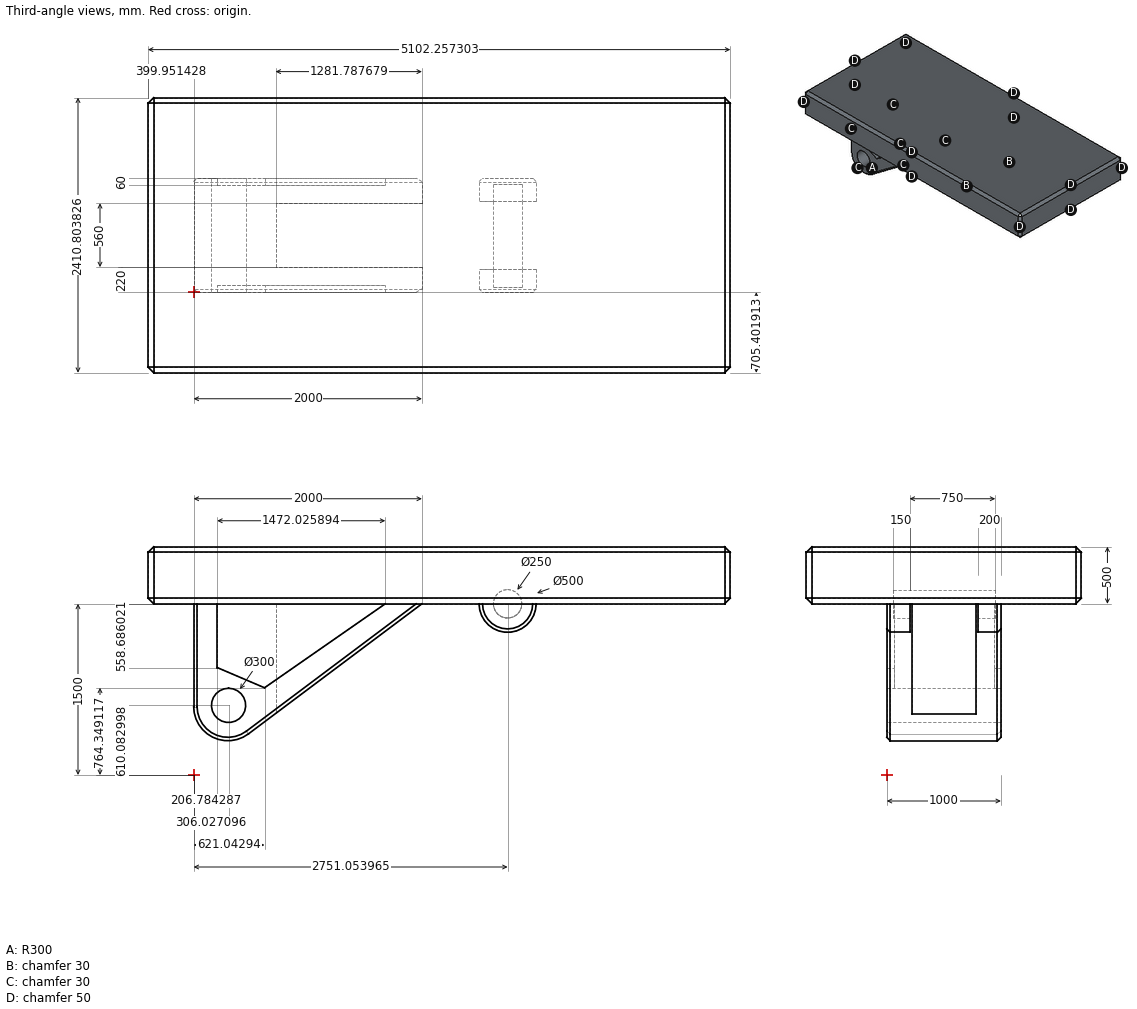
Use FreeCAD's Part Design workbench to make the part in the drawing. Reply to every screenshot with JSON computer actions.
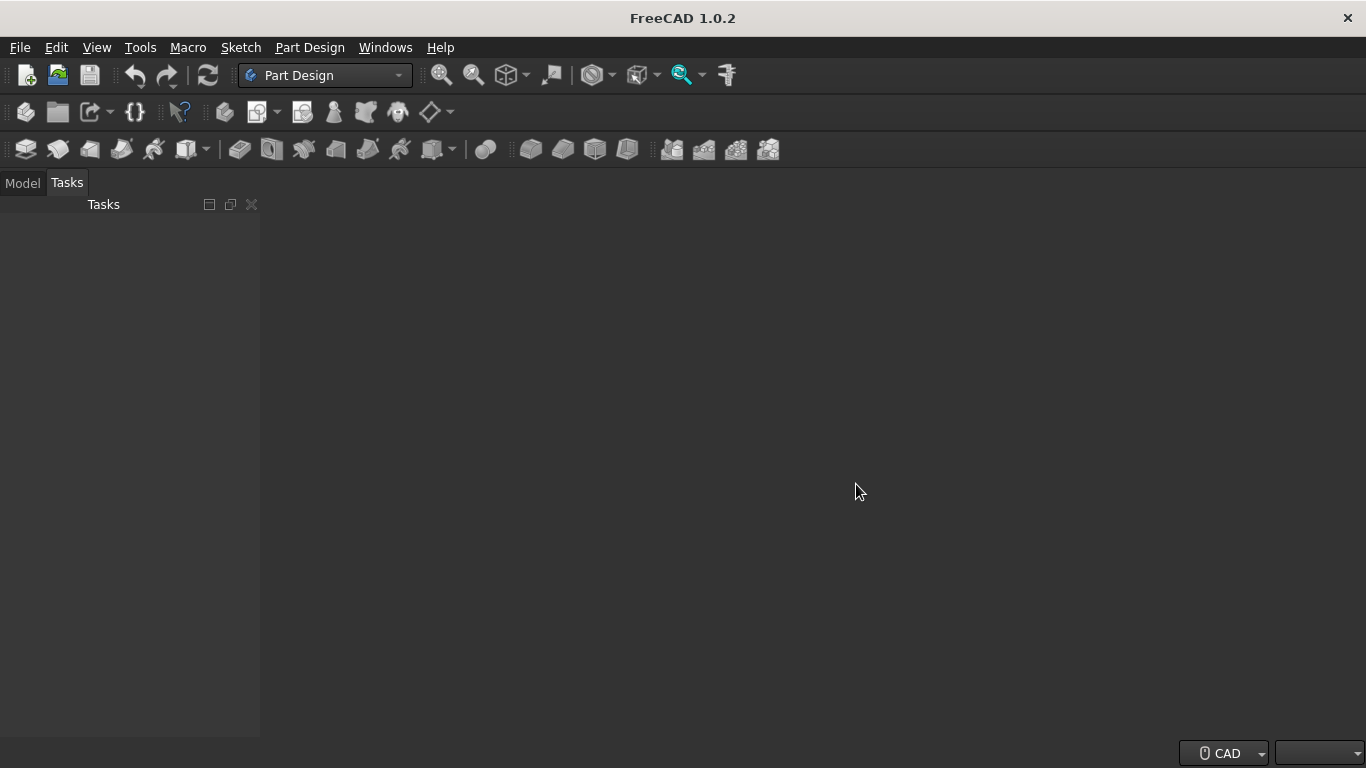
{"action": "left_click", "coordinate": [26, 76]}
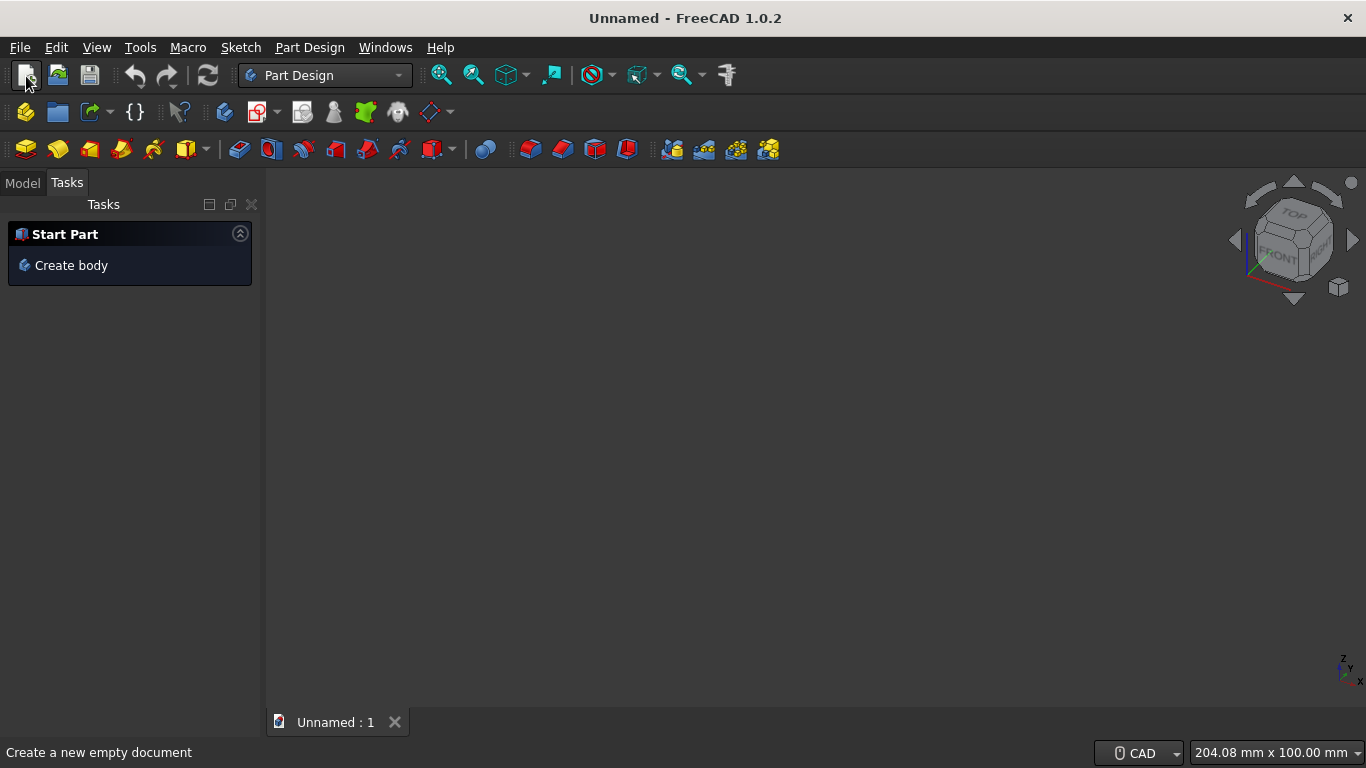
{"action": "left_click", "coordinate": [258, 112]}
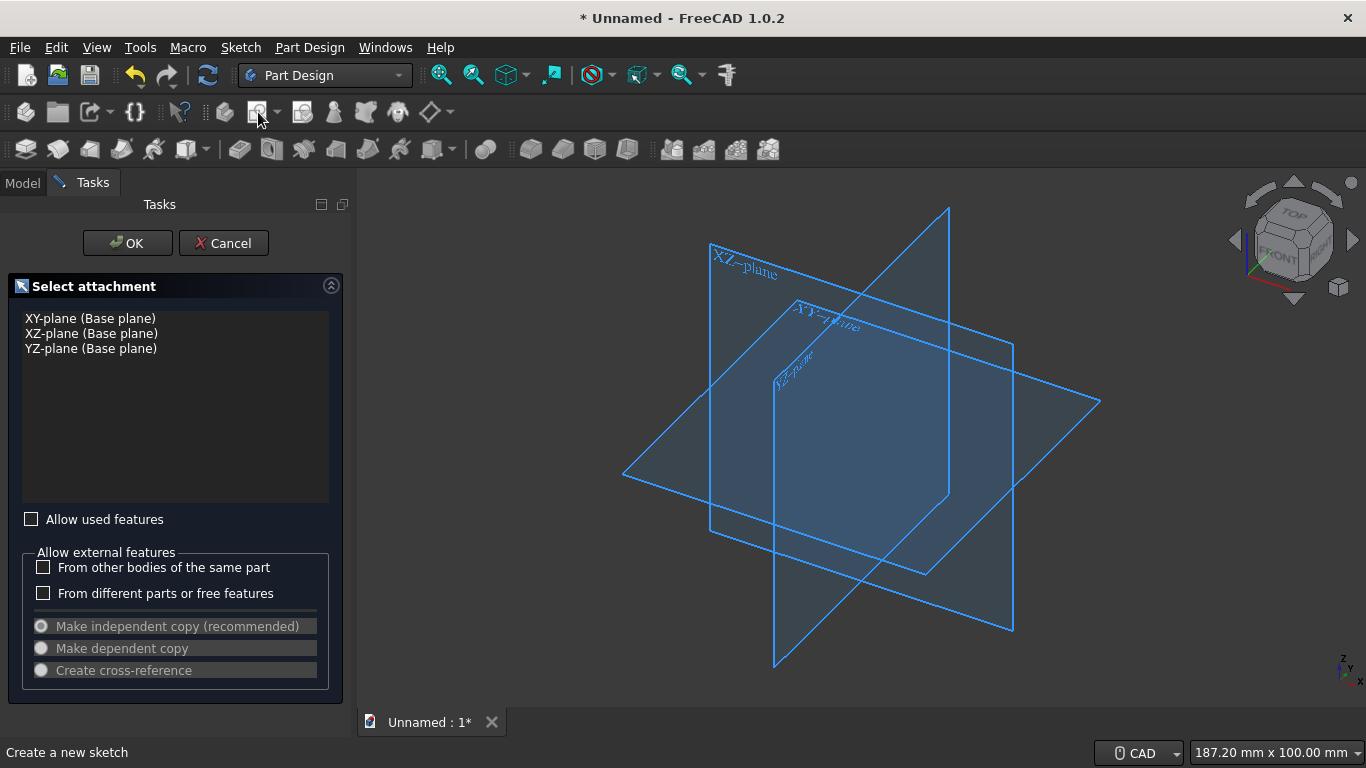
{"action": "left_click", "coordinate": [82, 334]}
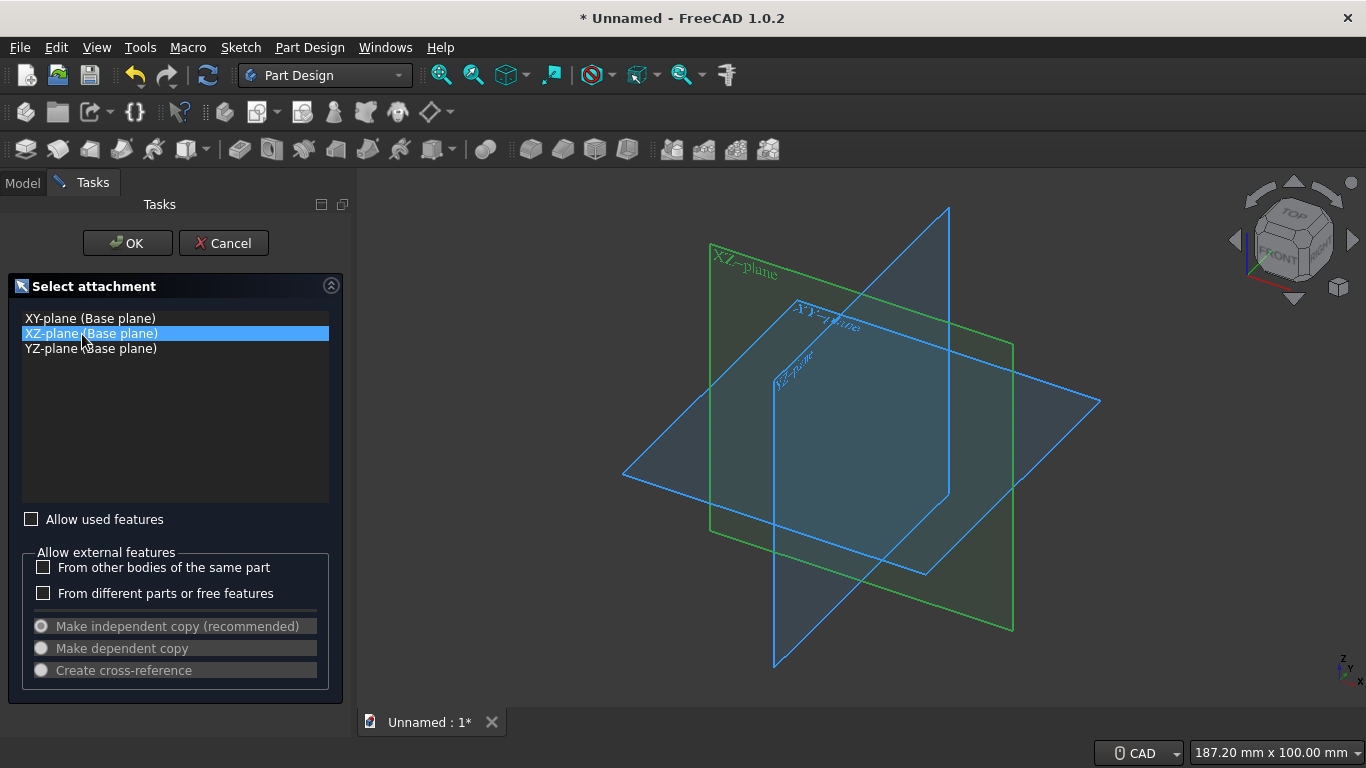
{"action": "left_click", "coordinate": [128, 243]}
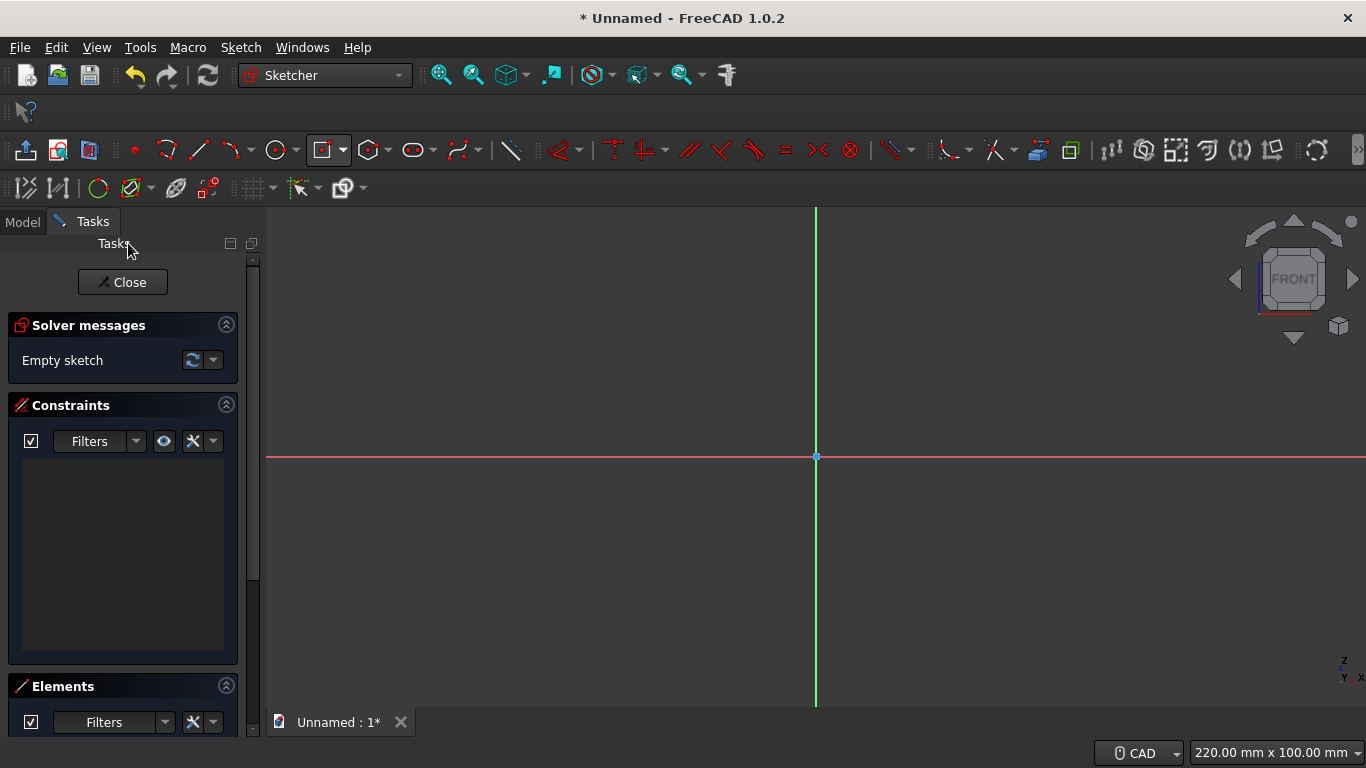
{"action": "scroll", "coordinate": [482, 653], "scroll_direction": "down", "scroll_amount": 15}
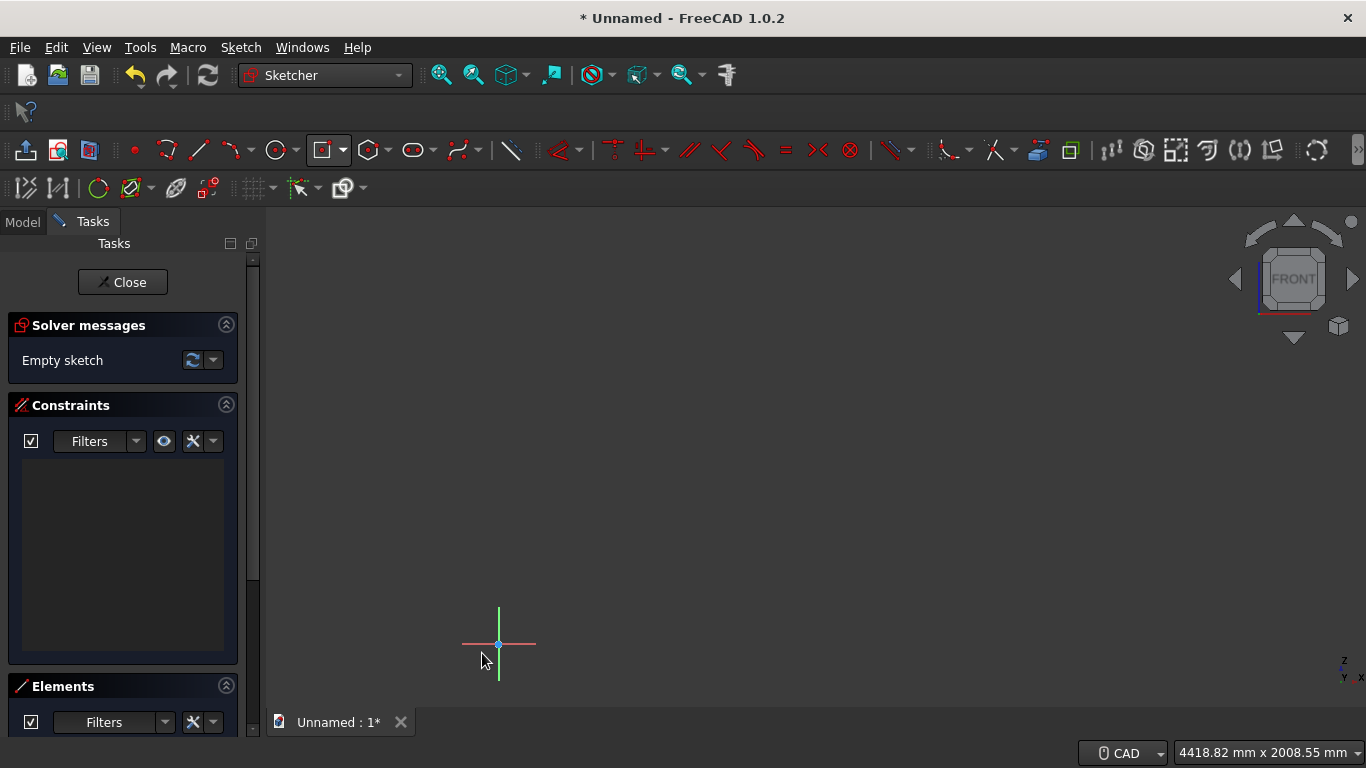
{"action": "left_click", "coordinate": [168, 150]}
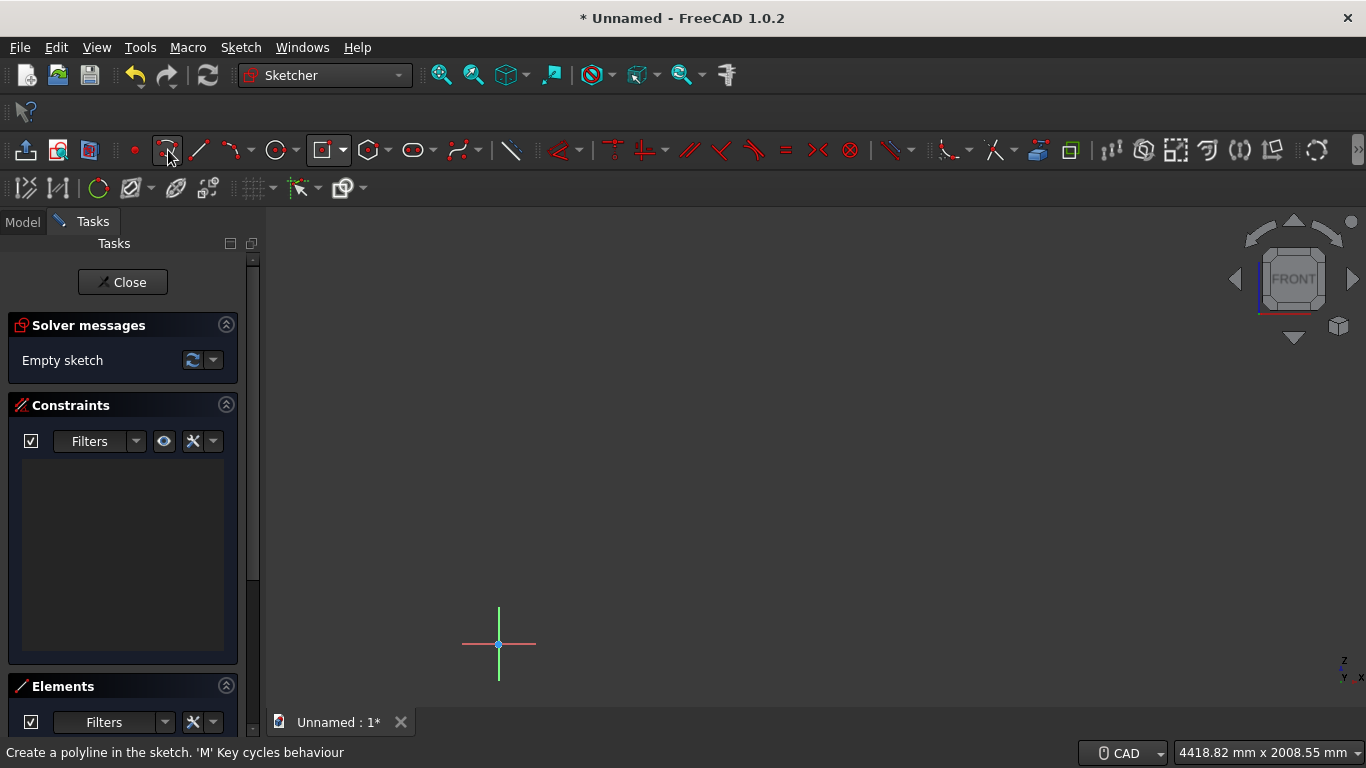
{"action": "left_click", "coordinate": [499, 644]}
{"action": "left_click", "coordinate": [508, 271]}
{"action": "left_click", "coordinate": [997, 271]}
{"action": "left_click", "coordinate": [499, 644]}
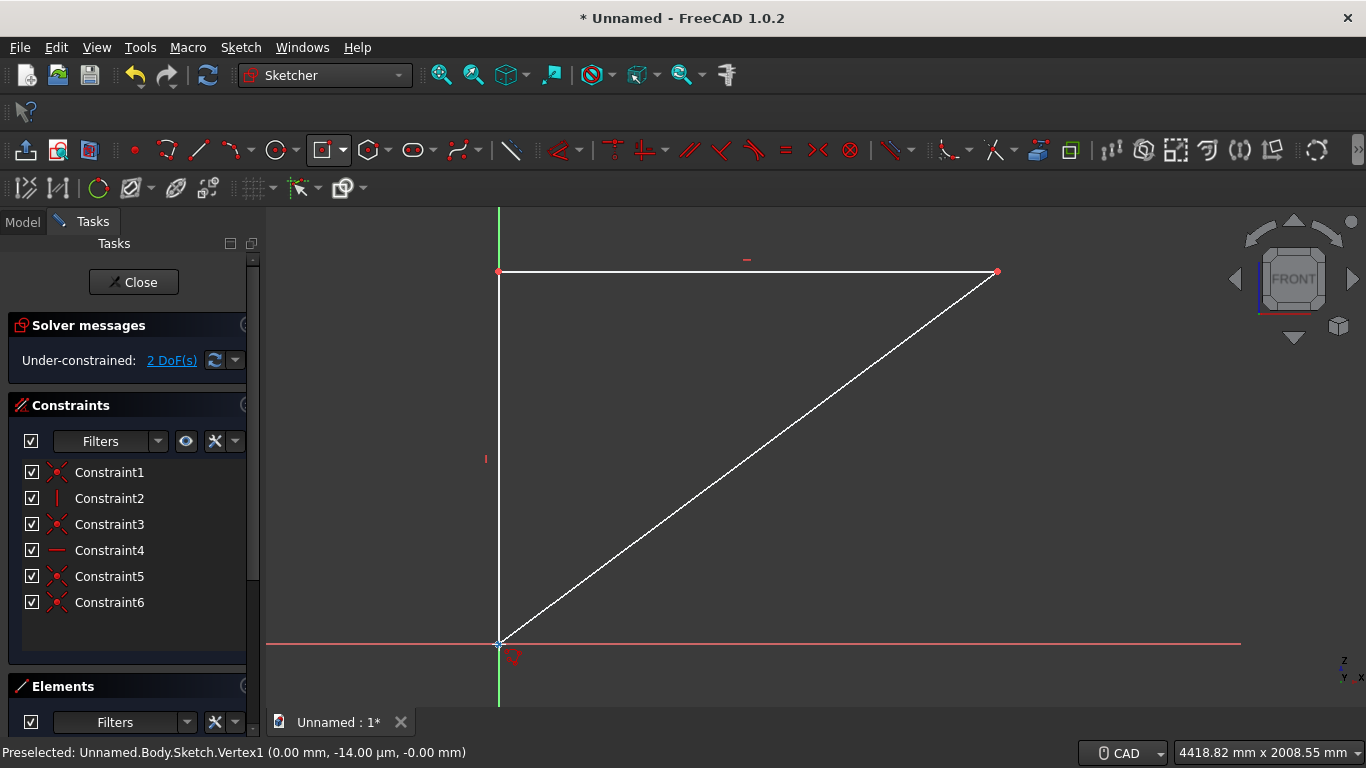
{"action": "key", "text": "g c"}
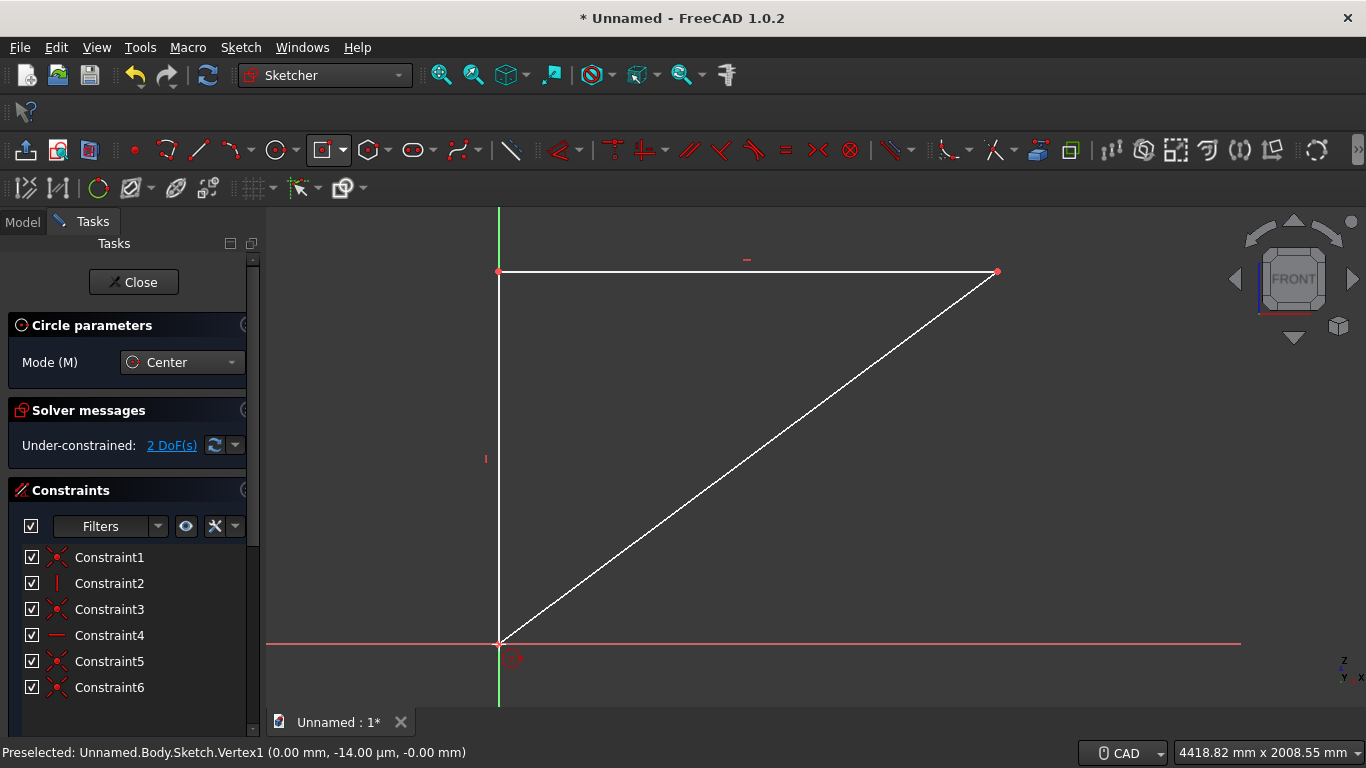
{"action": "left_click", "coordinate": [575, 492]}
{"action": "mouse_move", "coordinate": [601, 466]}